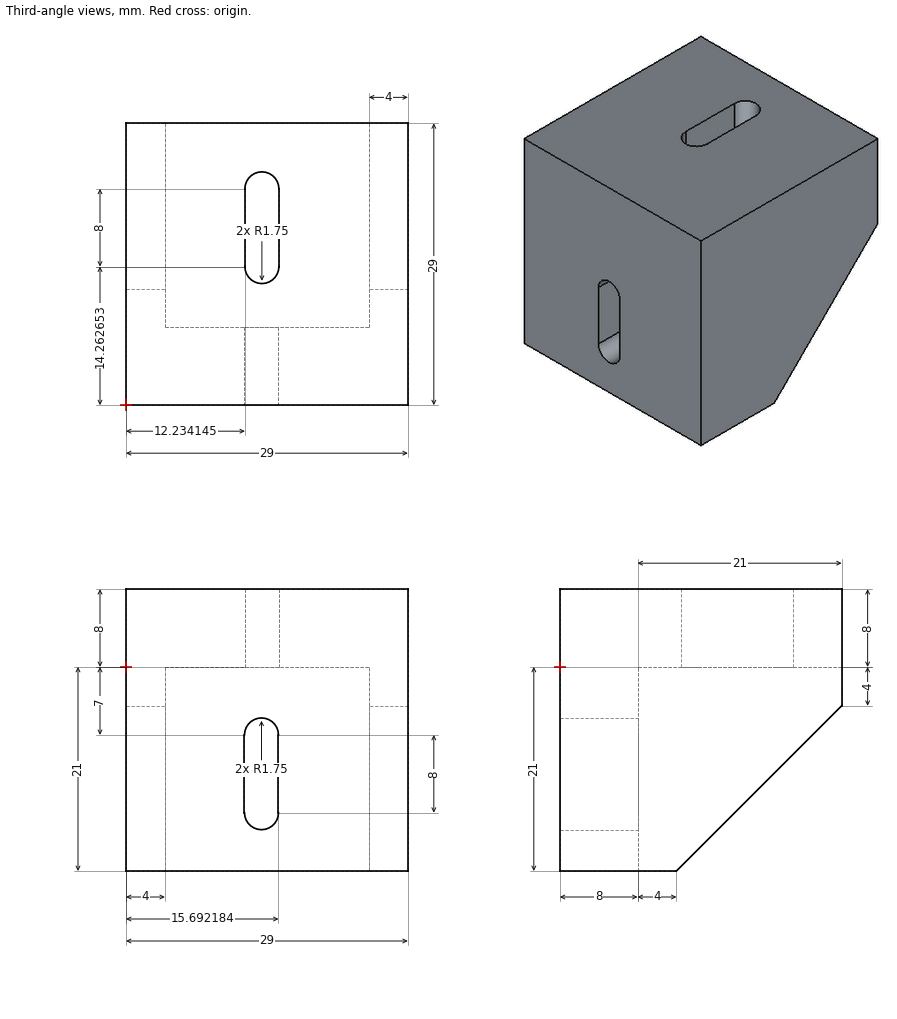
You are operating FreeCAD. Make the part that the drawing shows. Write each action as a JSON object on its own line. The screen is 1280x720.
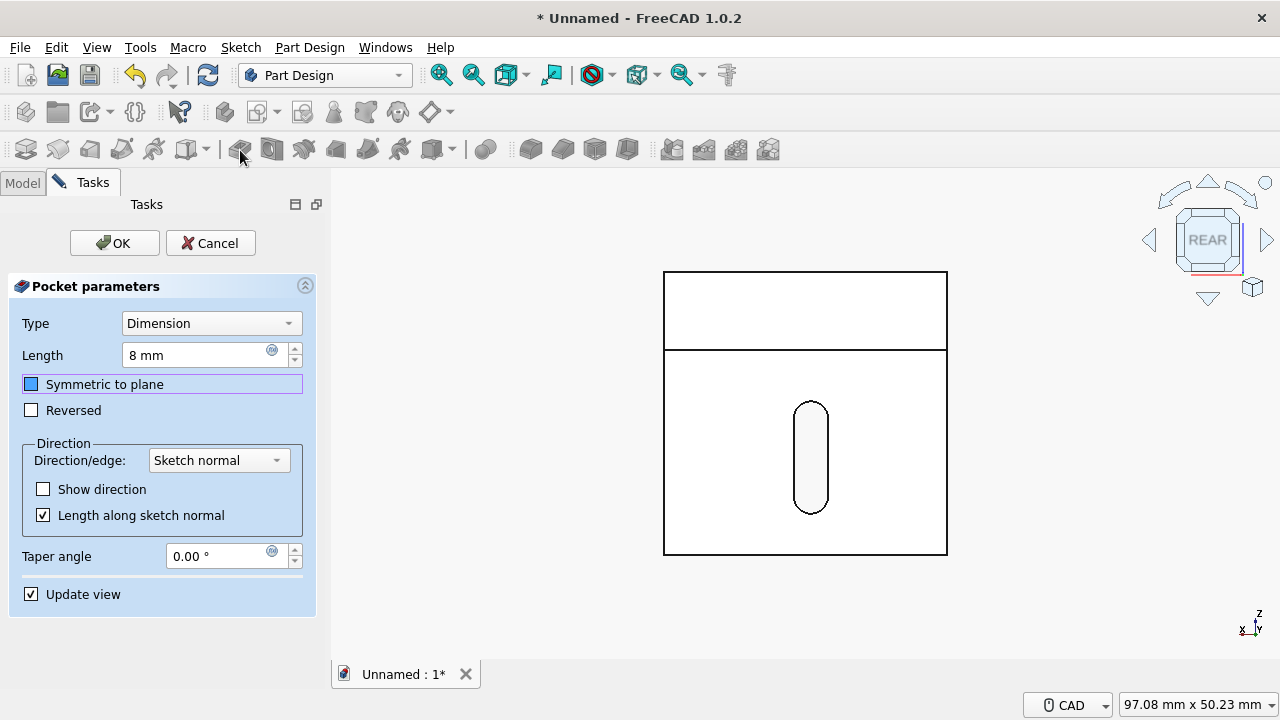
{"action": "left_click", "coordinate": [115, 243]}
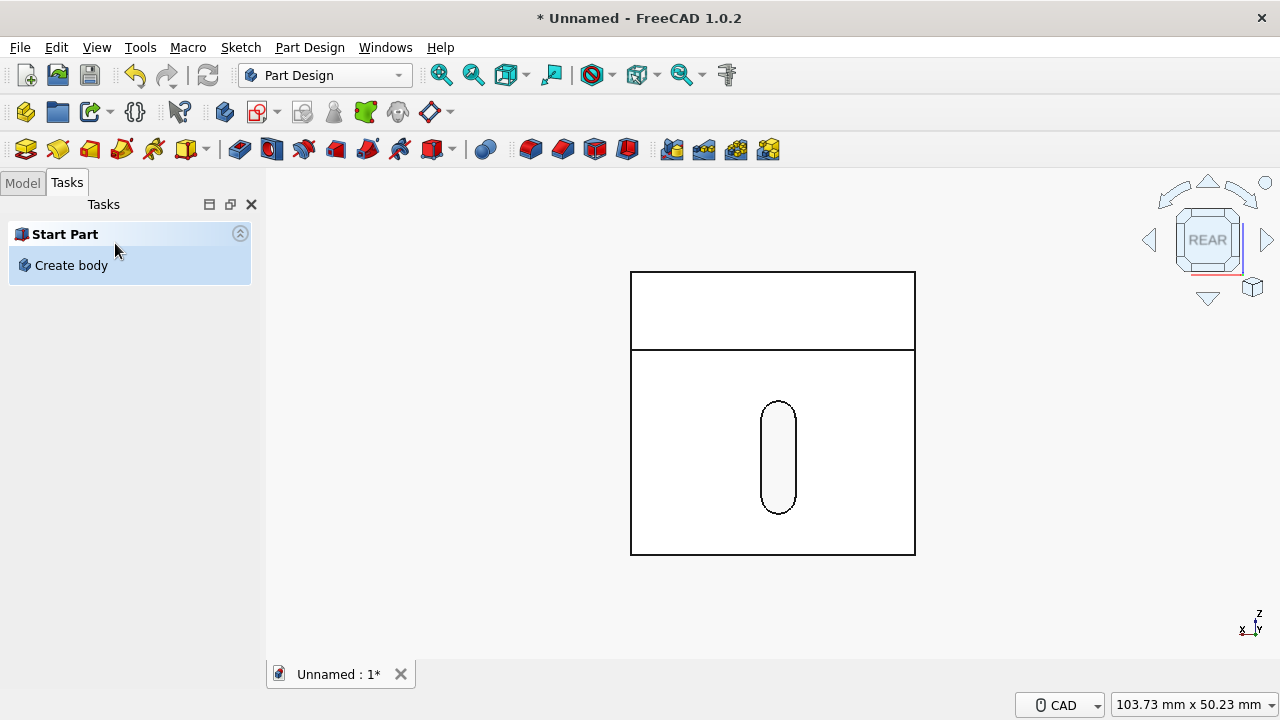
{"action": "key", "text": "0"}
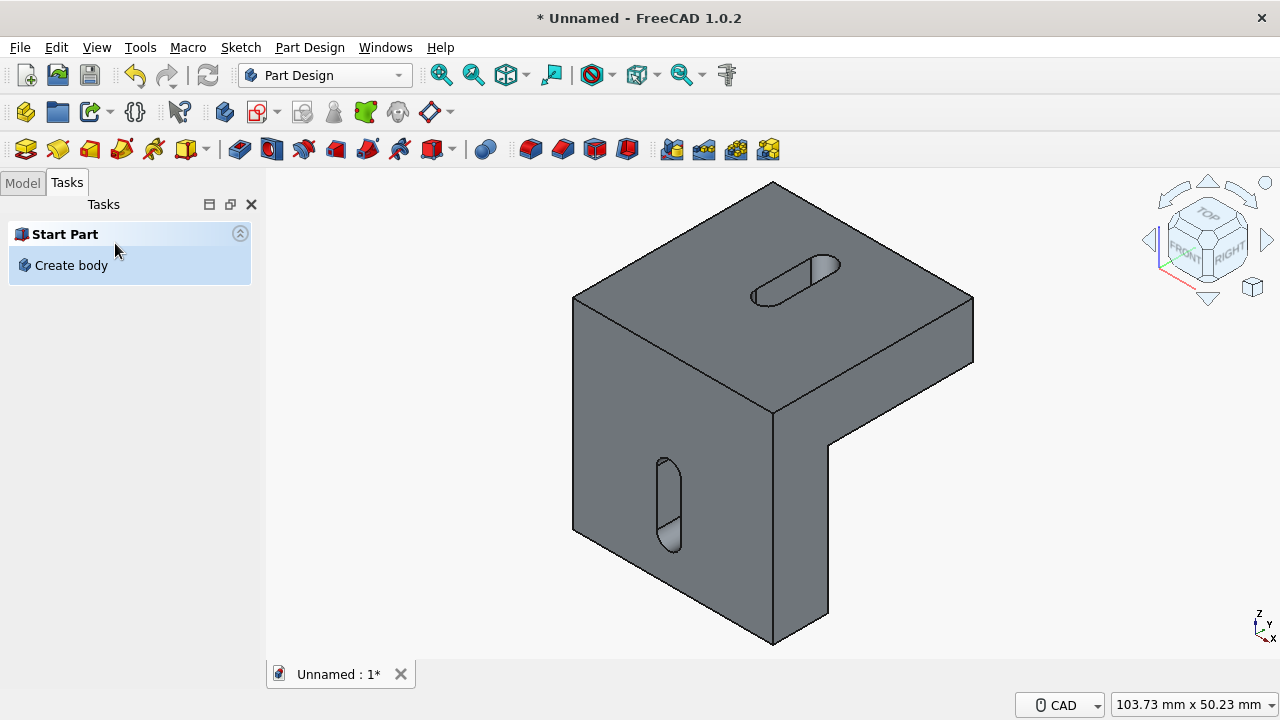
{"action": "left_click", "coordinate": [816, 437]}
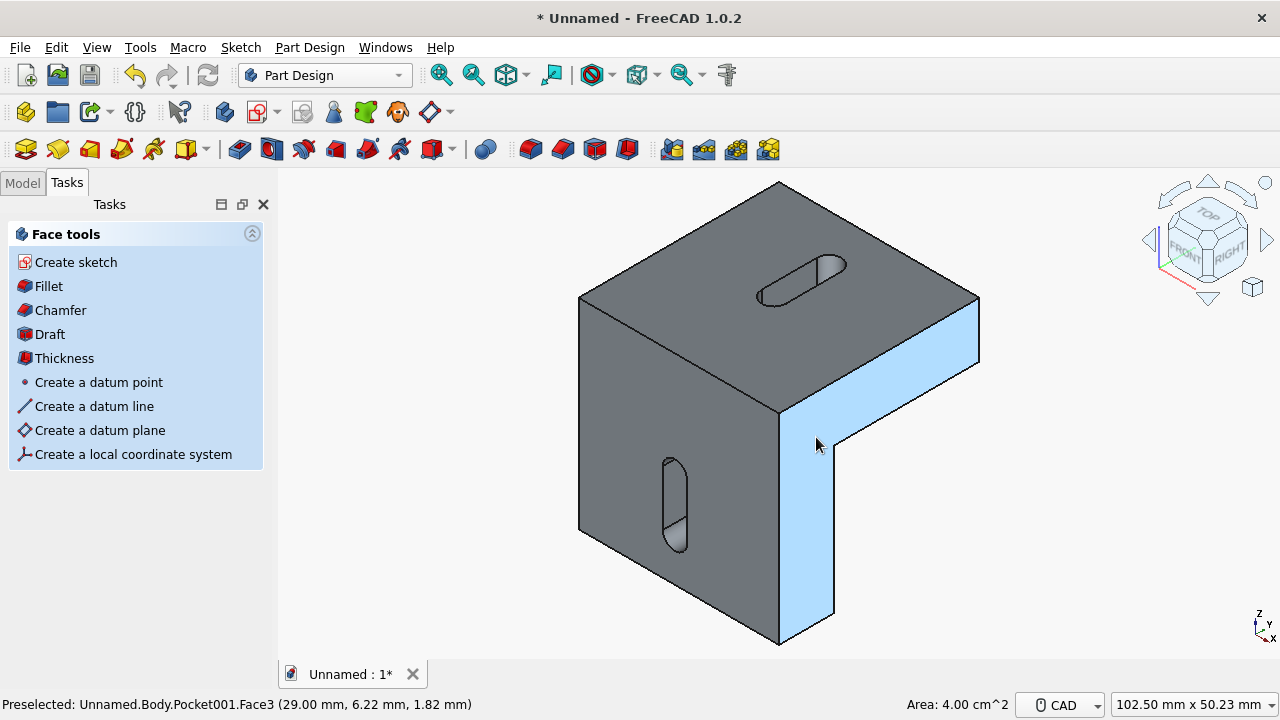
{"action": "left_click", "coordinate": [258, 112]}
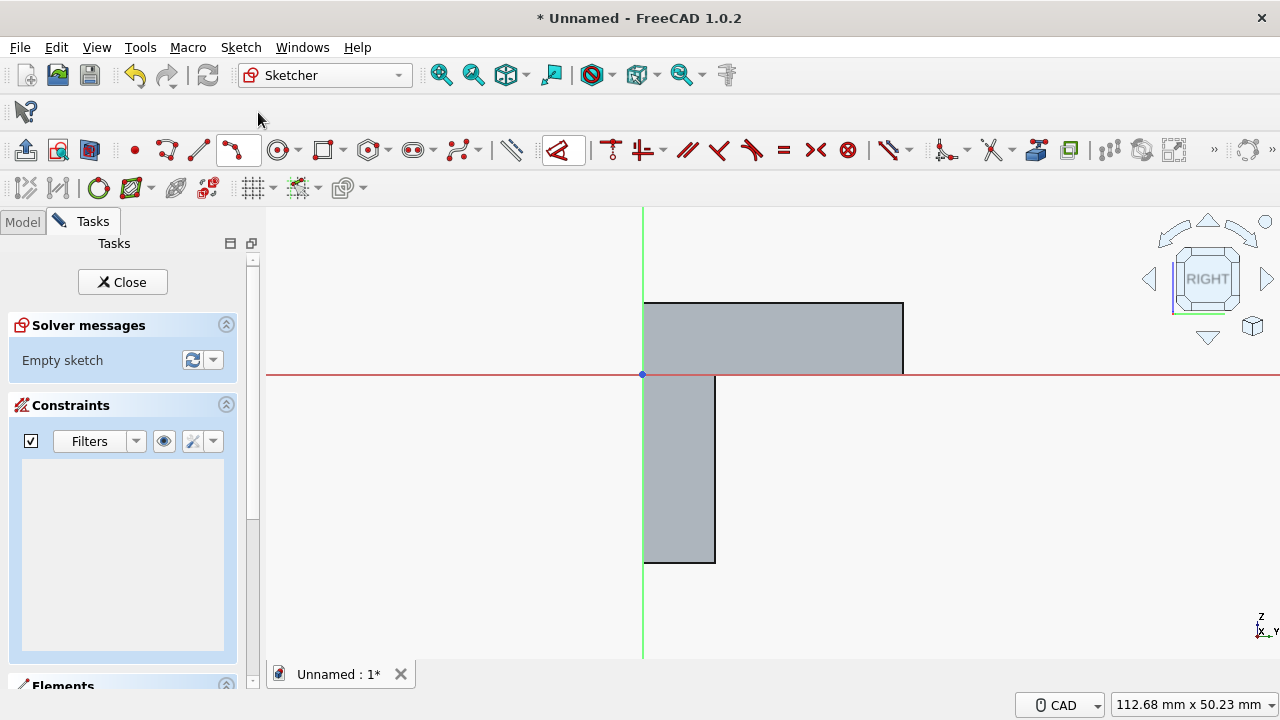
{"action": "scroll", "coordinate": [912, 542], "scroll_direction": "up", "scroll_amount": 2}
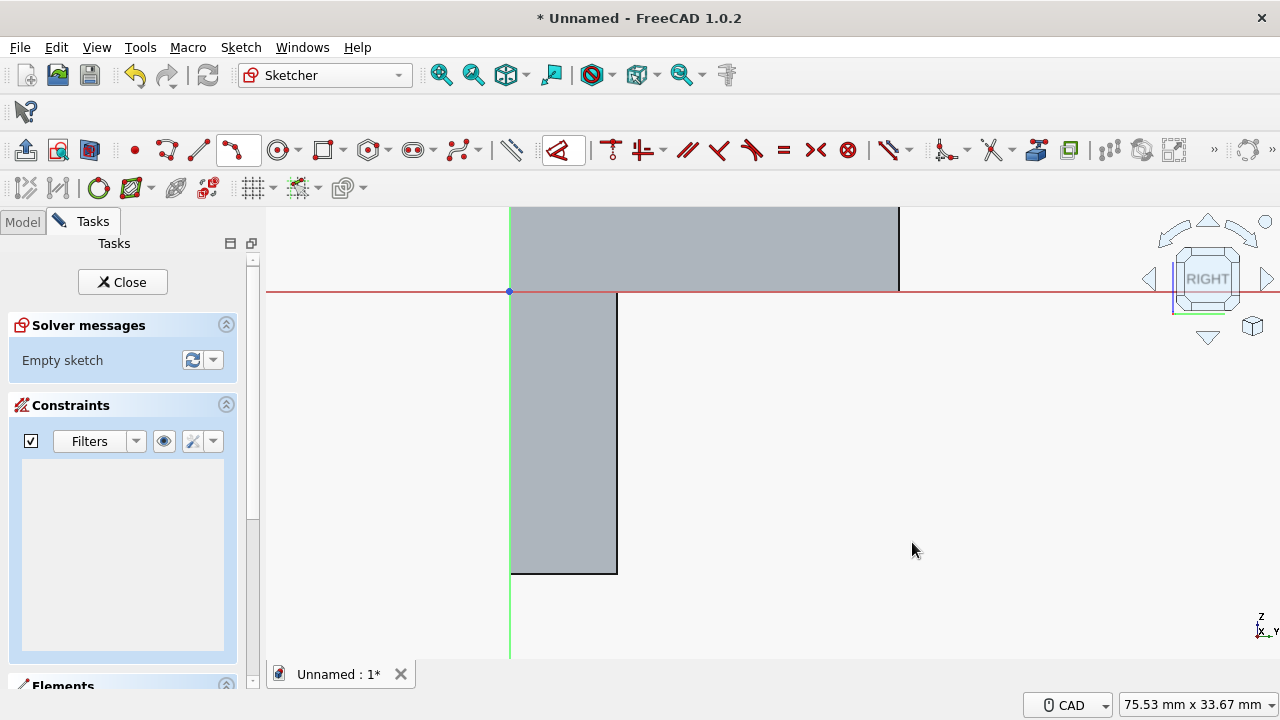
{"action": "key", "text": "g m"}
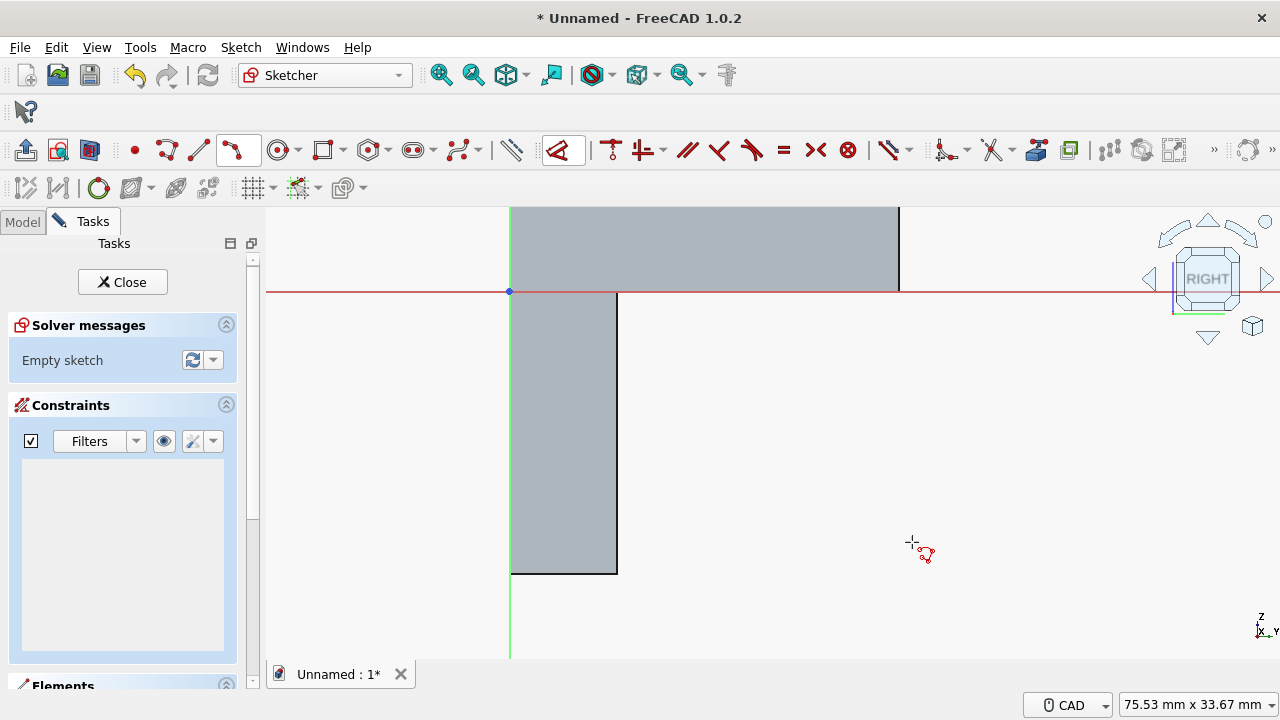
{"action": "left_click", "coordinate": [617, 292]}
{"action": "left_click", "coordinate": [617, 574]}
{"action": "left_click", "coordinate": [671, 574]}
{"action": "left_click", "coordinate": [899, 345]}
{"action": "left_click", "coordinate": [899, 301]}
{"action": "left_click", "coordinate": [617, 292]}
{"action": "key", "text": "Escape"}
{"action": "key", "text": "Escape"}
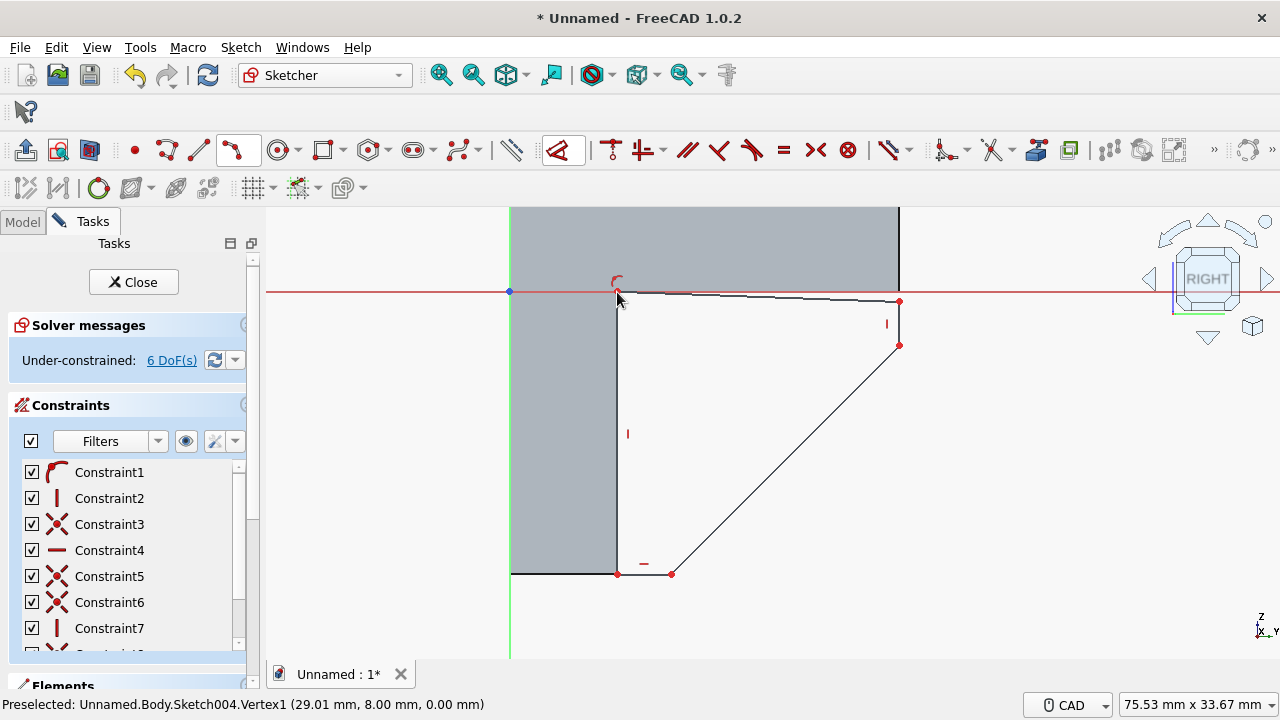
{"action": "left_click", "coordinate": [702, 295]}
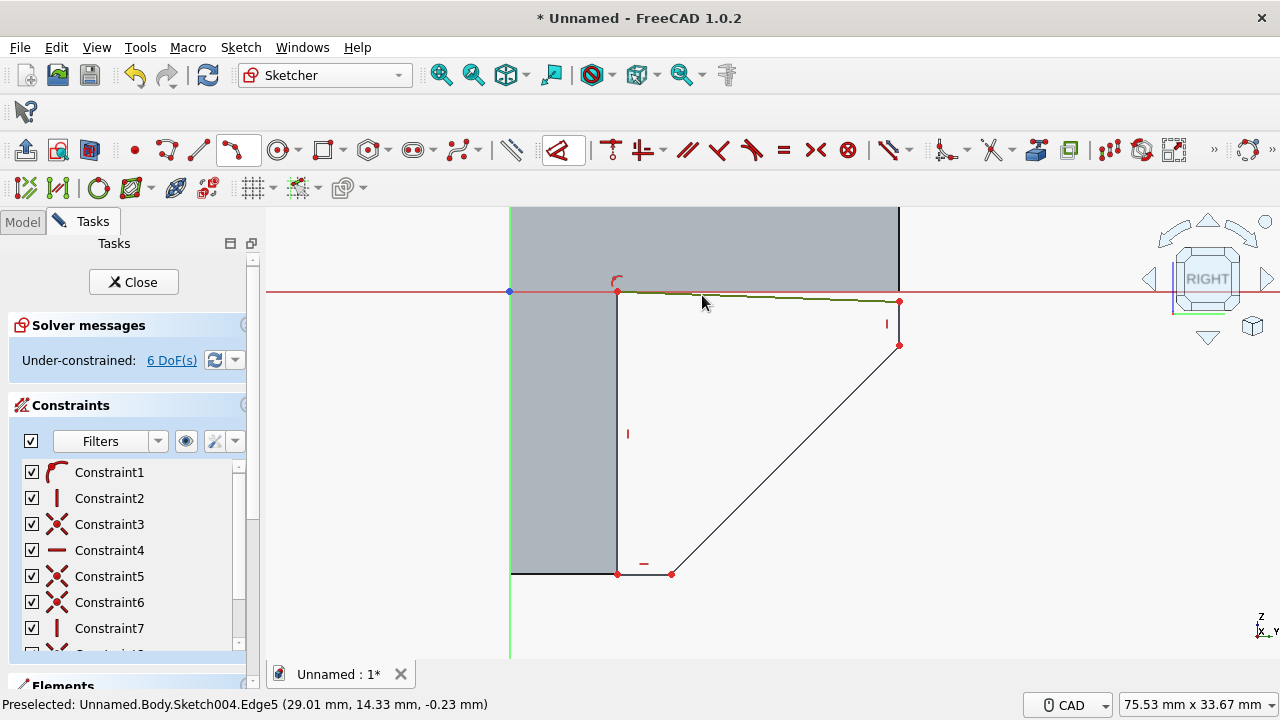
{"action": "left_click", "coordinate": [666, 150]}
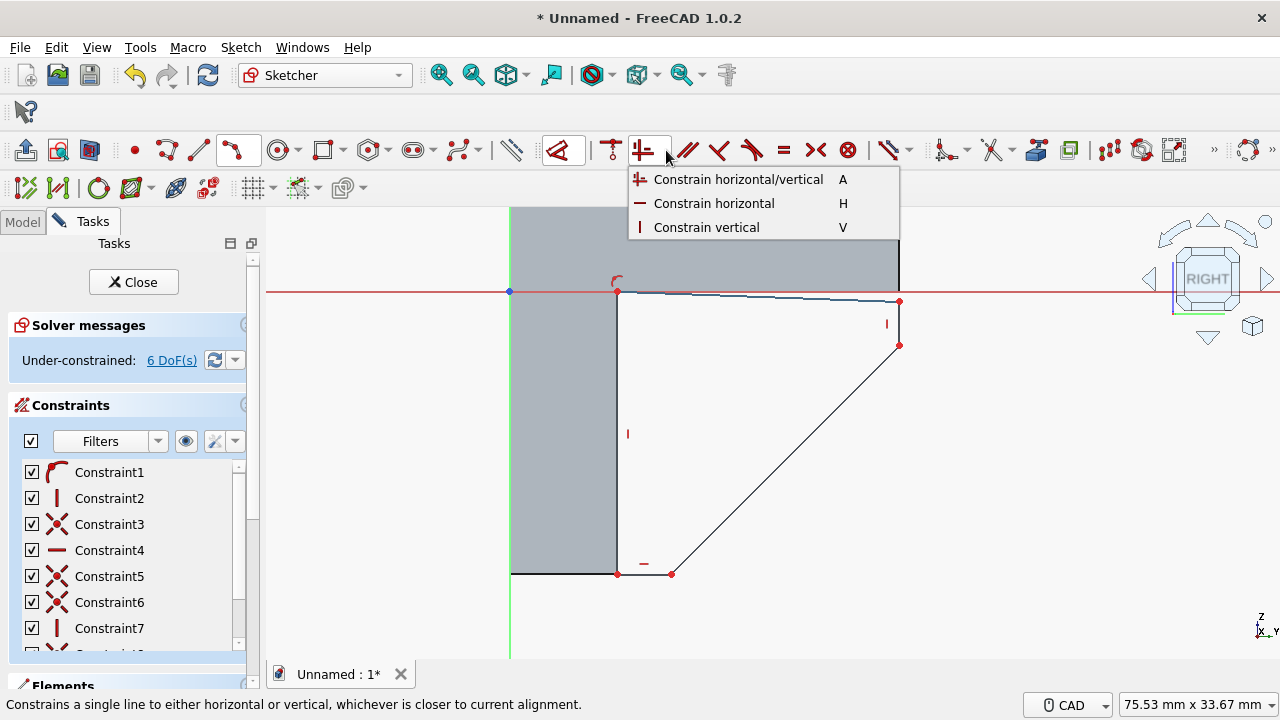
{"action": "left_click", "coordinate": [764, 203]}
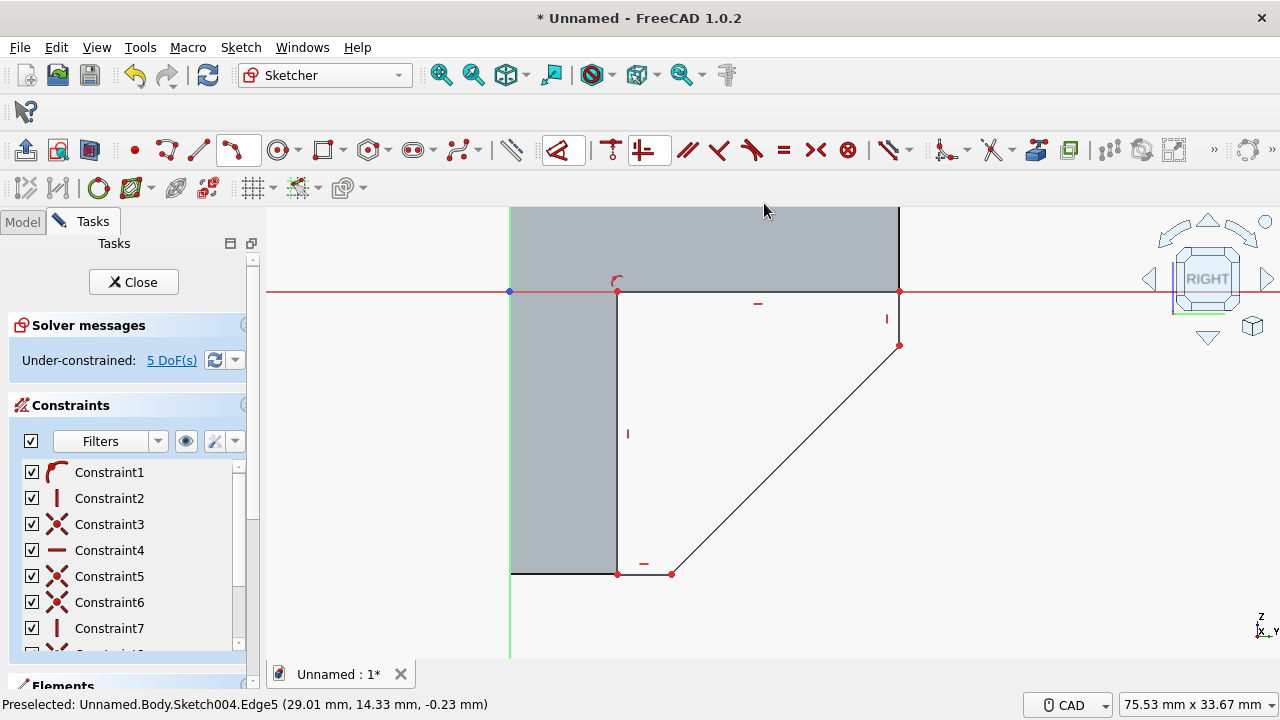
{"action": "left_click", "coordinate": [633, 575]}